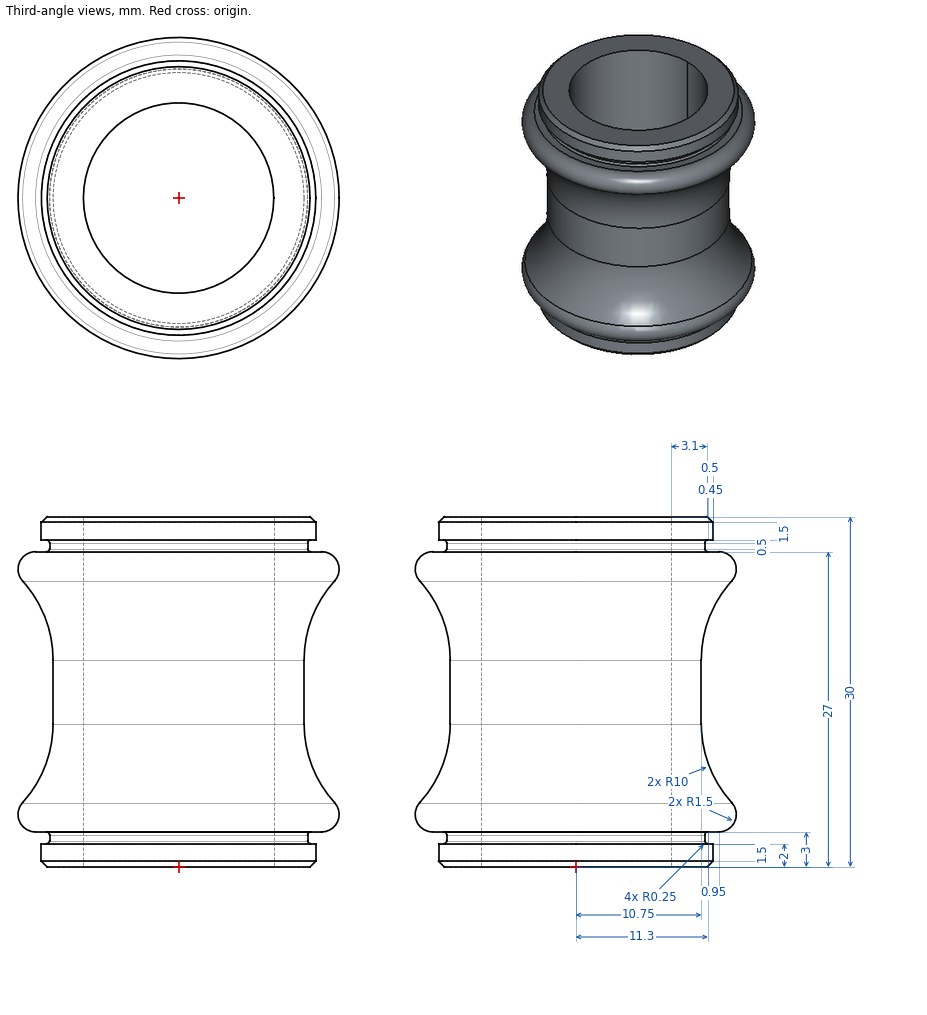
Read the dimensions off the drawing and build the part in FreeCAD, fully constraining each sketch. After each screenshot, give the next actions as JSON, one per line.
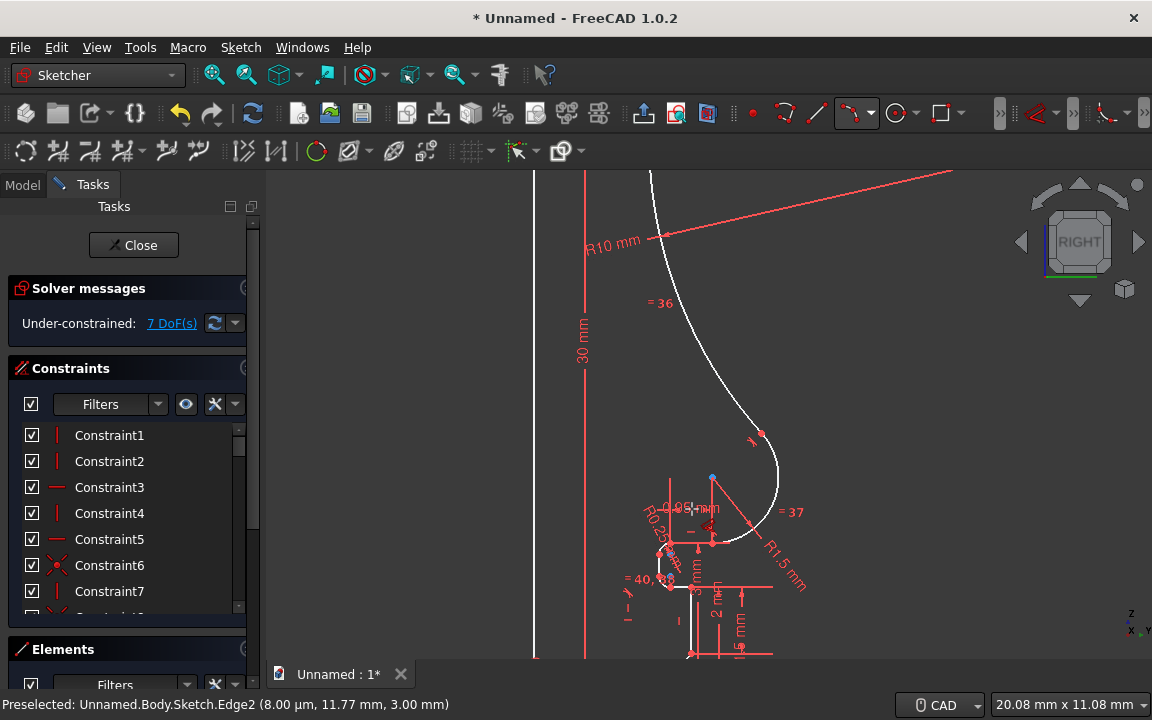
{"action": "scroll", "coordinate": [695, 546], "scroll_direction": "down", "scroll_amount": 7}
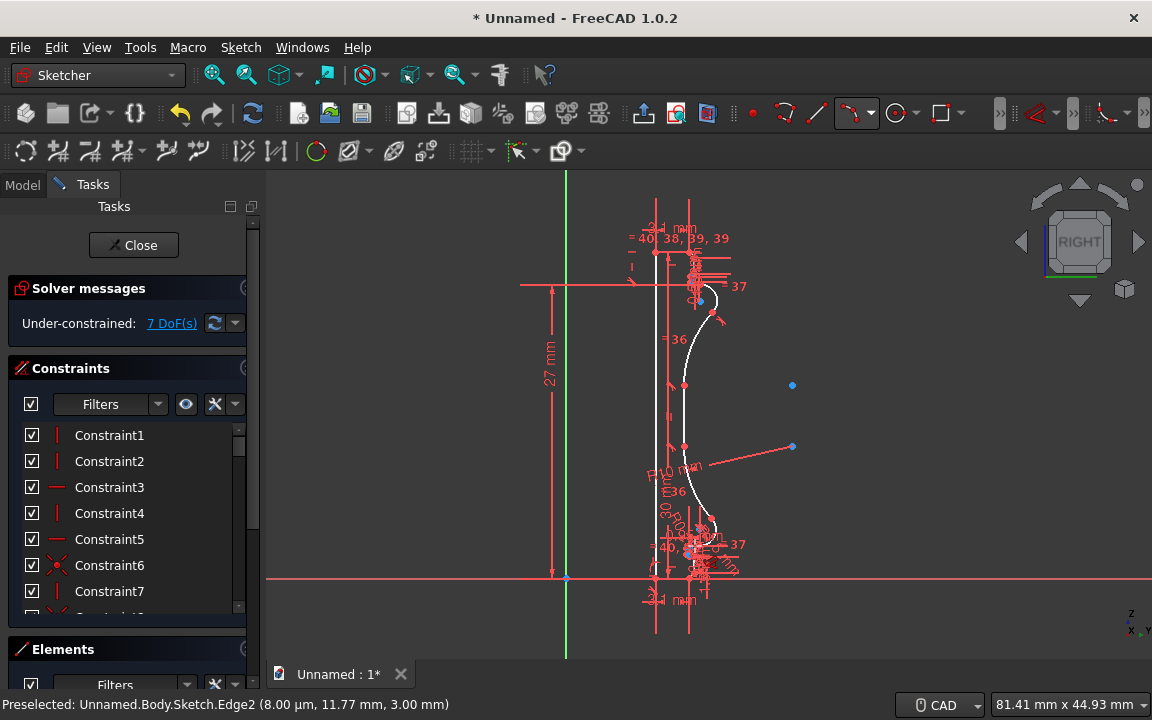
{"action": "scroll", "coordinate": [699, 285], "scroll_direction": "up", "scroll_amount": 10}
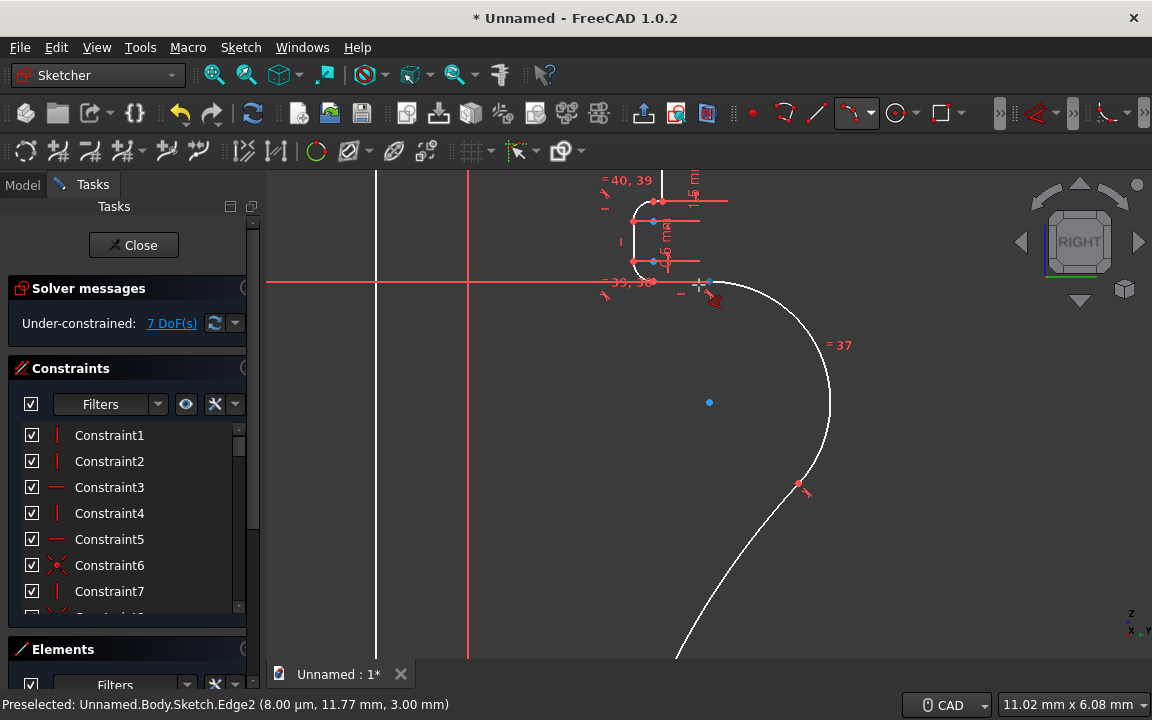
{"action": "left_click", "coordinate": [693, 282]}
{"action": "left_click", "coordinate": [682, 316]}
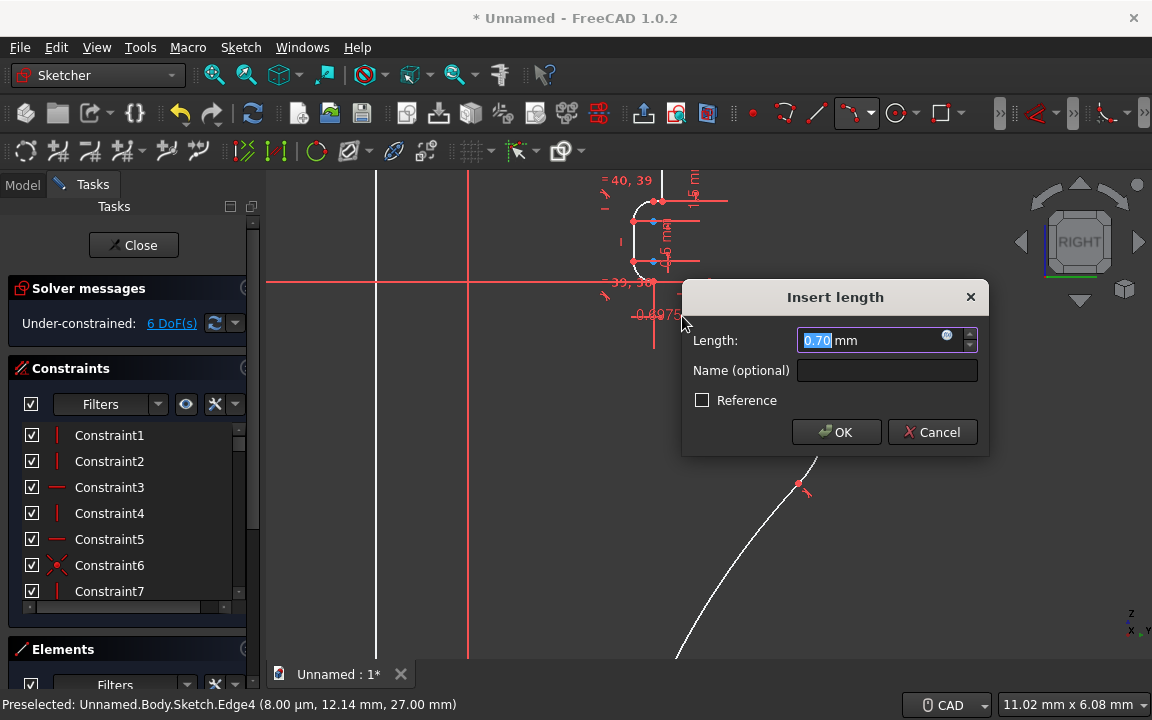
{"action": "type", "text": "0.95"}
{"action": "key", "text": "Return"}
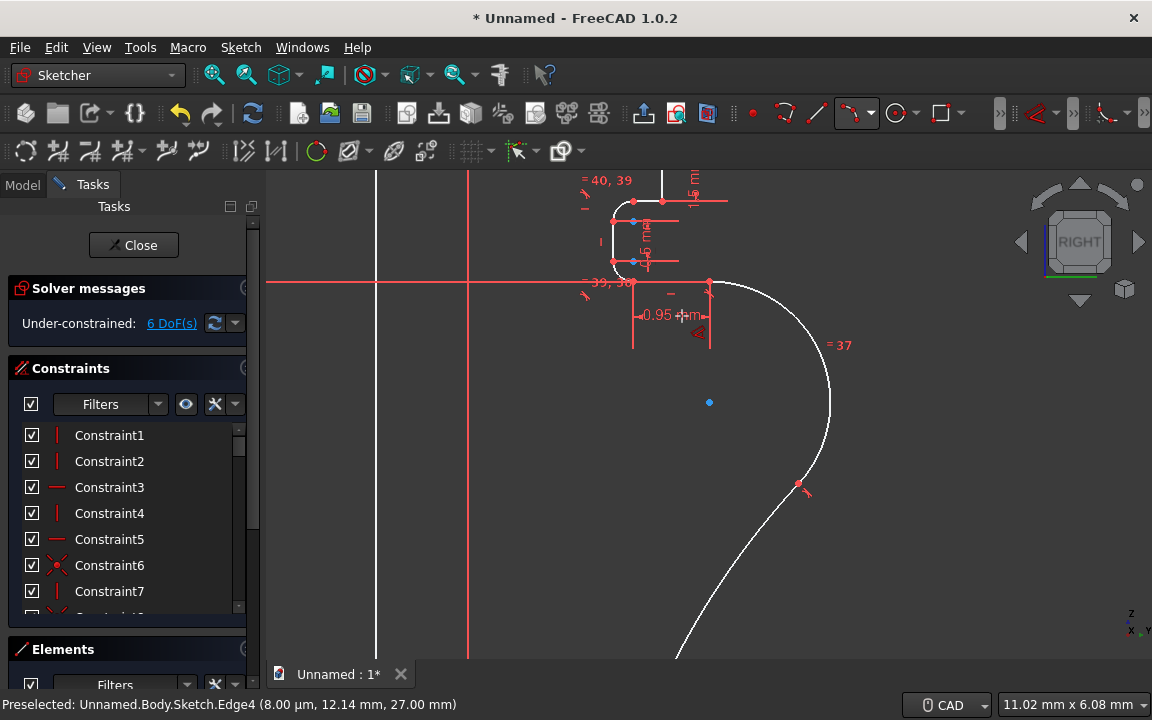
{"action": "left_click", "coordinate": [645, 201]}
{"action": "left_click", "coordinate": [648, 355]}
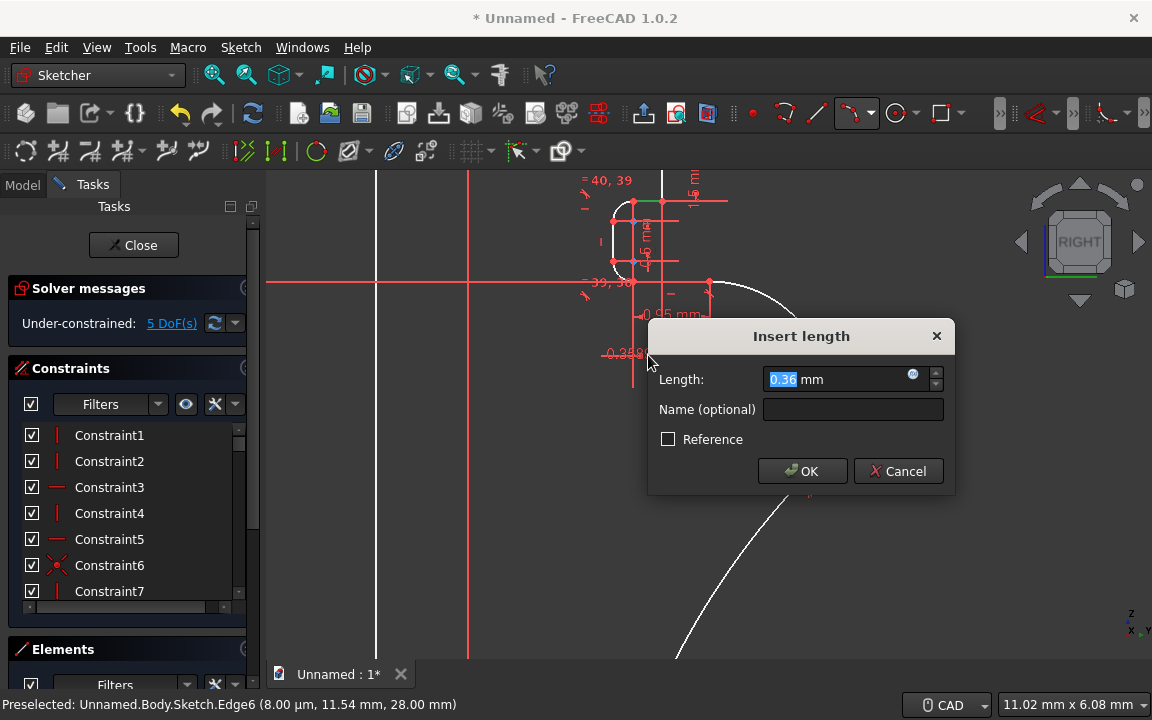
{"action": "type", "text": "0.45"}
{"action": "key", "text": "Return"}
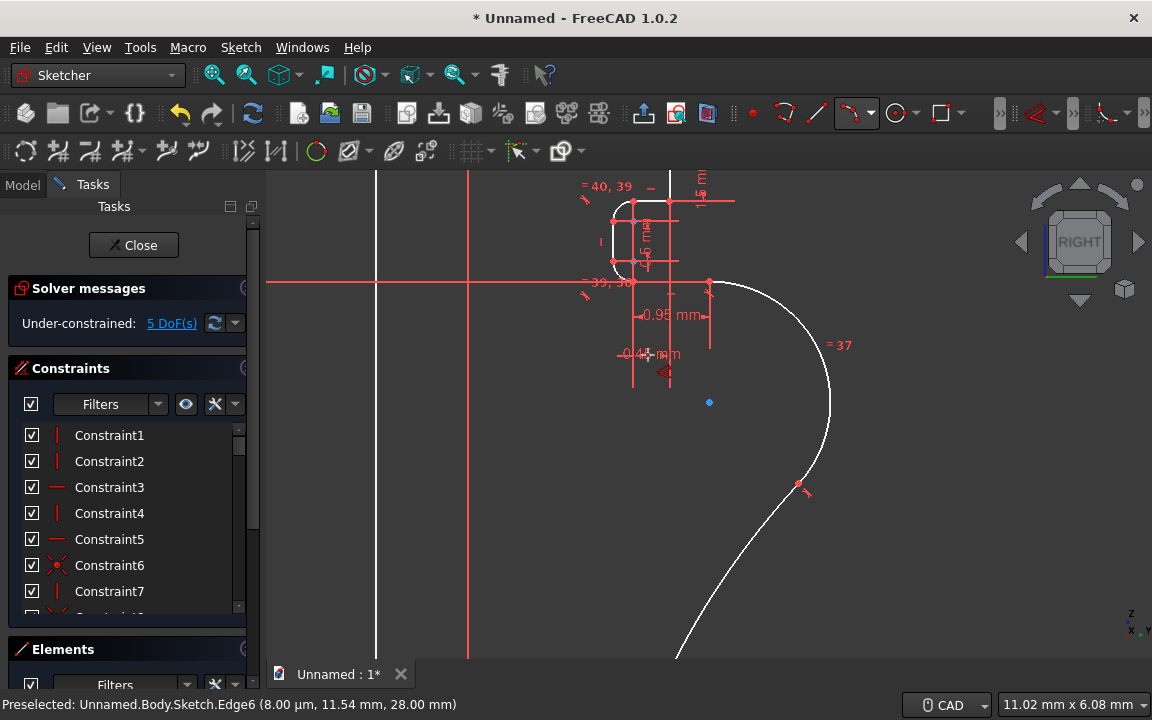
{"action": "scroll", "coordinate": [699, 284], "scroll_direction": "down", "scroll_amount": 10}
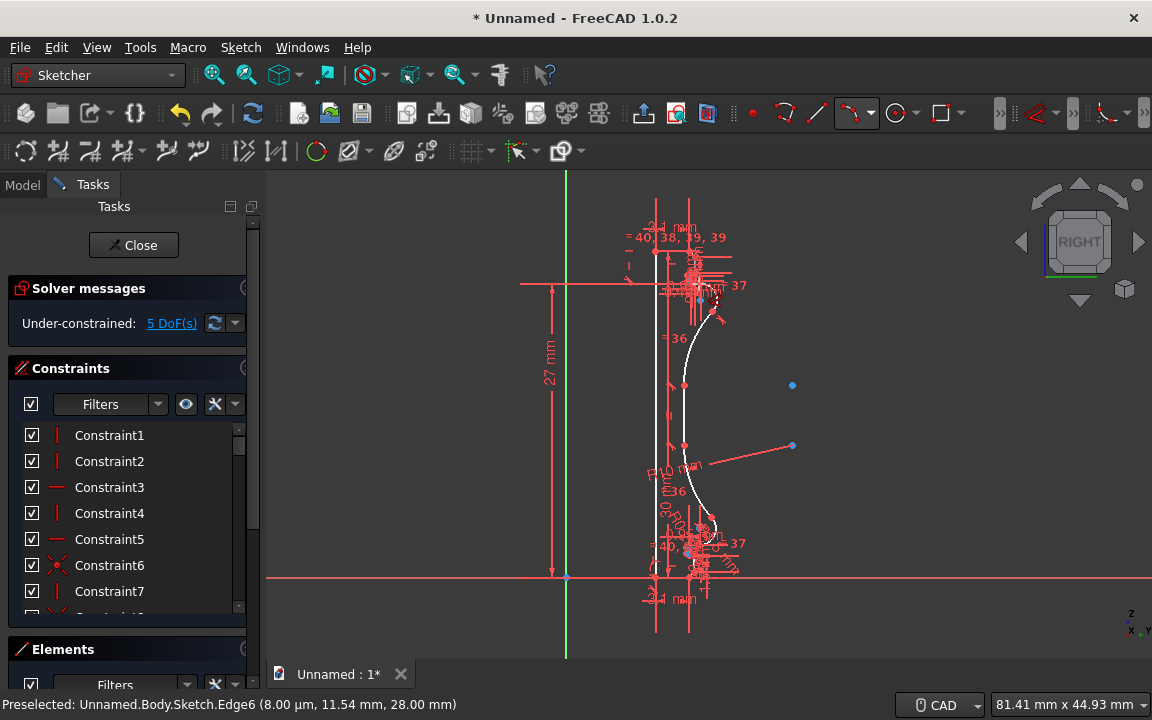
{"action": "scroll", "coordinate": [693, 556], "scroll_direction": "up", "scroll_amount": 11}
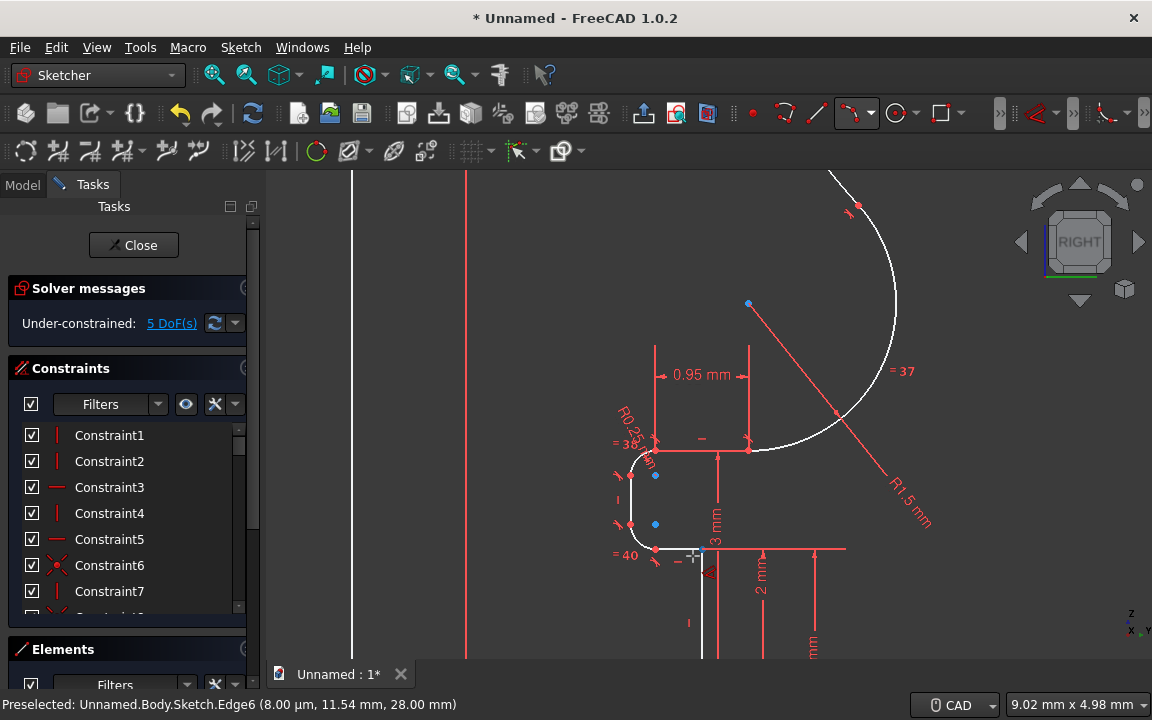
{"action": "left_click", "coordinate": [688, 549]}
{"action": "left_click", "coordinate": [679, 583]}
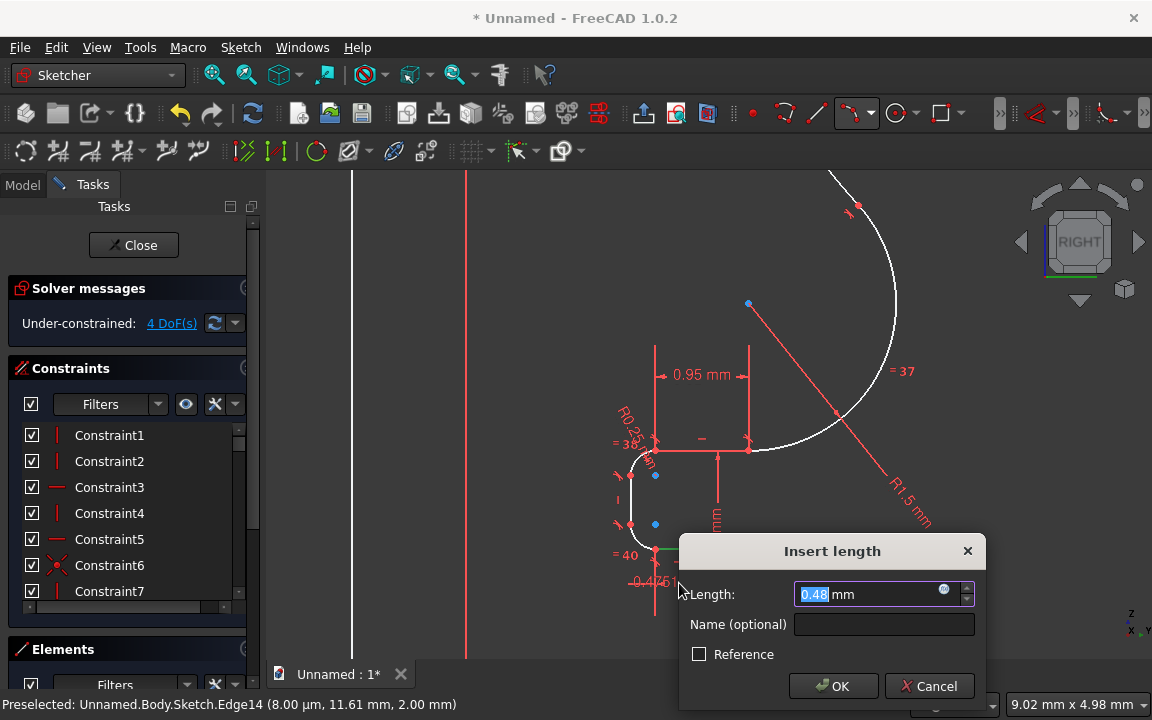
{"action": "type", "text": "0.45"}
{"action": "key", "text": "Return"}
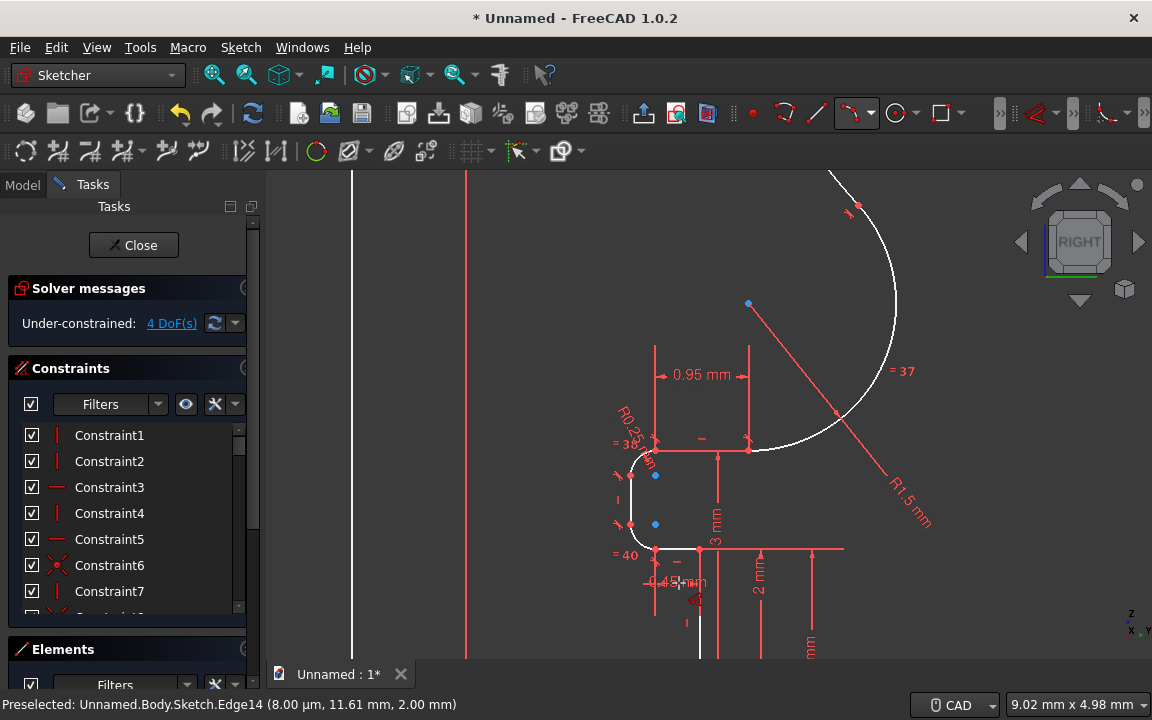
{"action": "scroll", "coordinate": [693, 557], "scroll_direction": "down", "scroll_amount": 11}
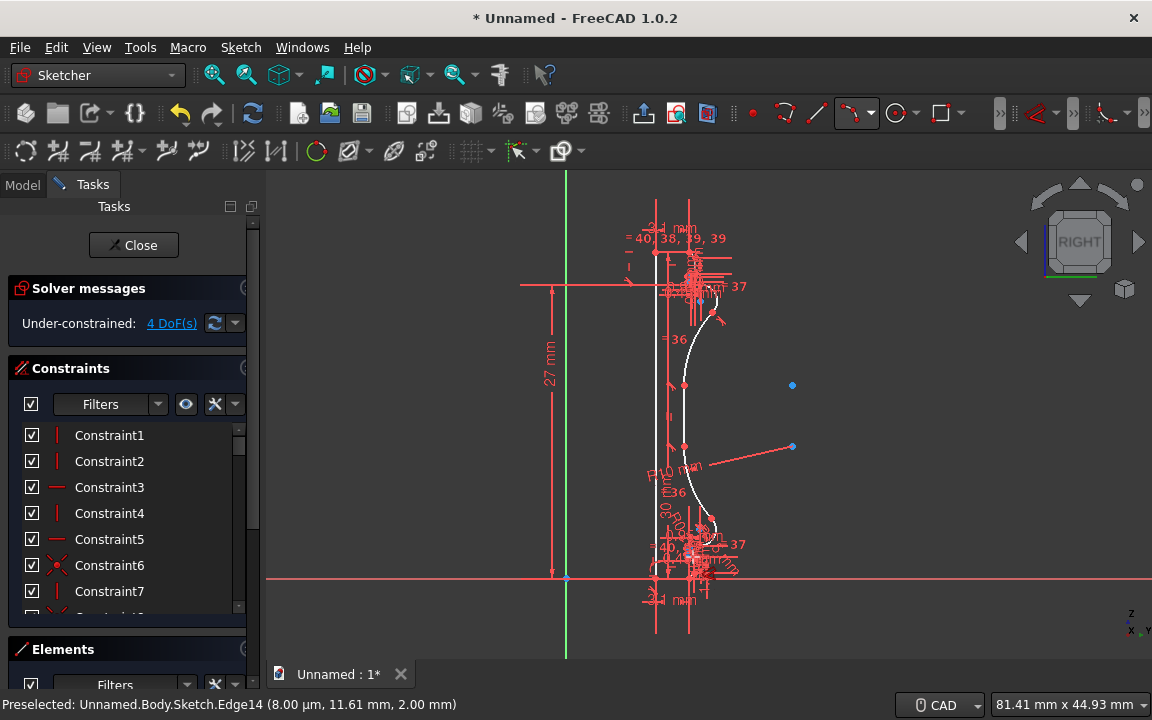
{"action": "scroll", "coordinate": [694, 256], "scroll_direction": "up", "scroll_amount": 10}